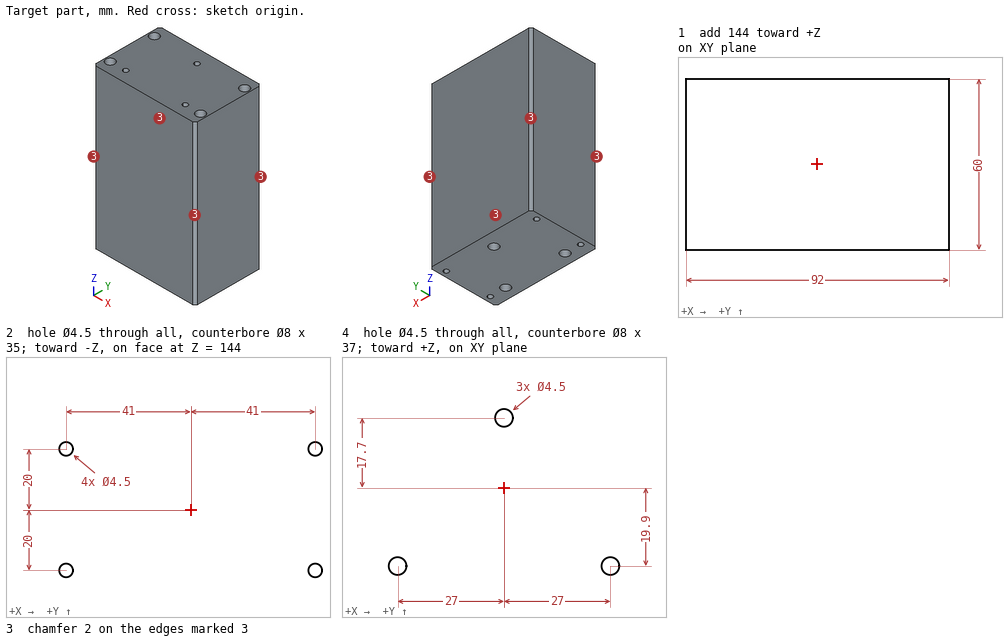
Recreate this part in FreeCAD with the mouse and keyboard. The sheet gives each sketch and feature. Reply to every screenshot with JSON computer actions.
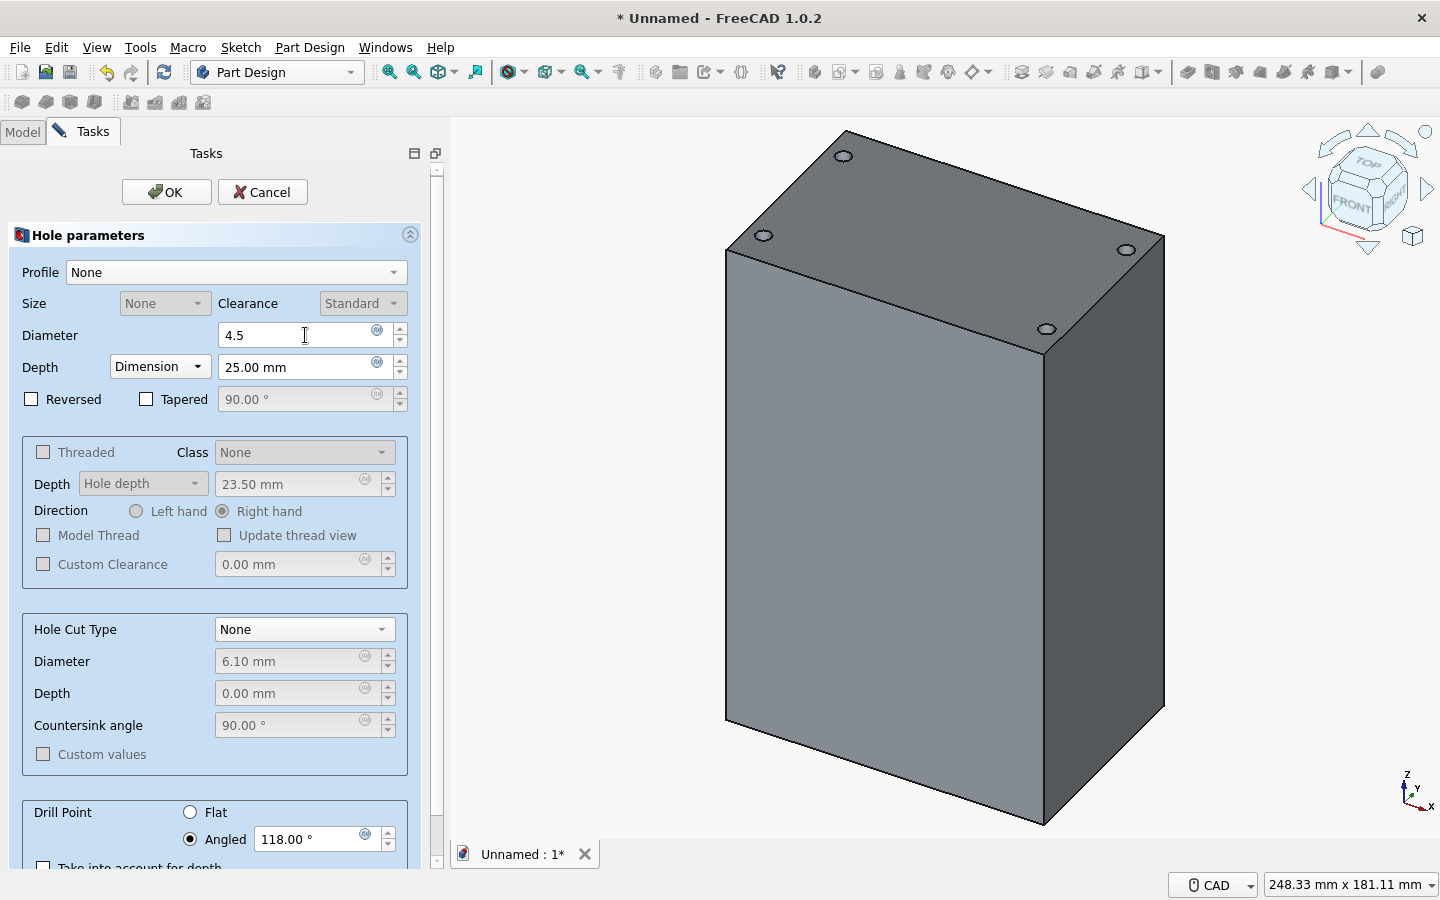
{"action": "left_click", "coordinate": [161, 366]}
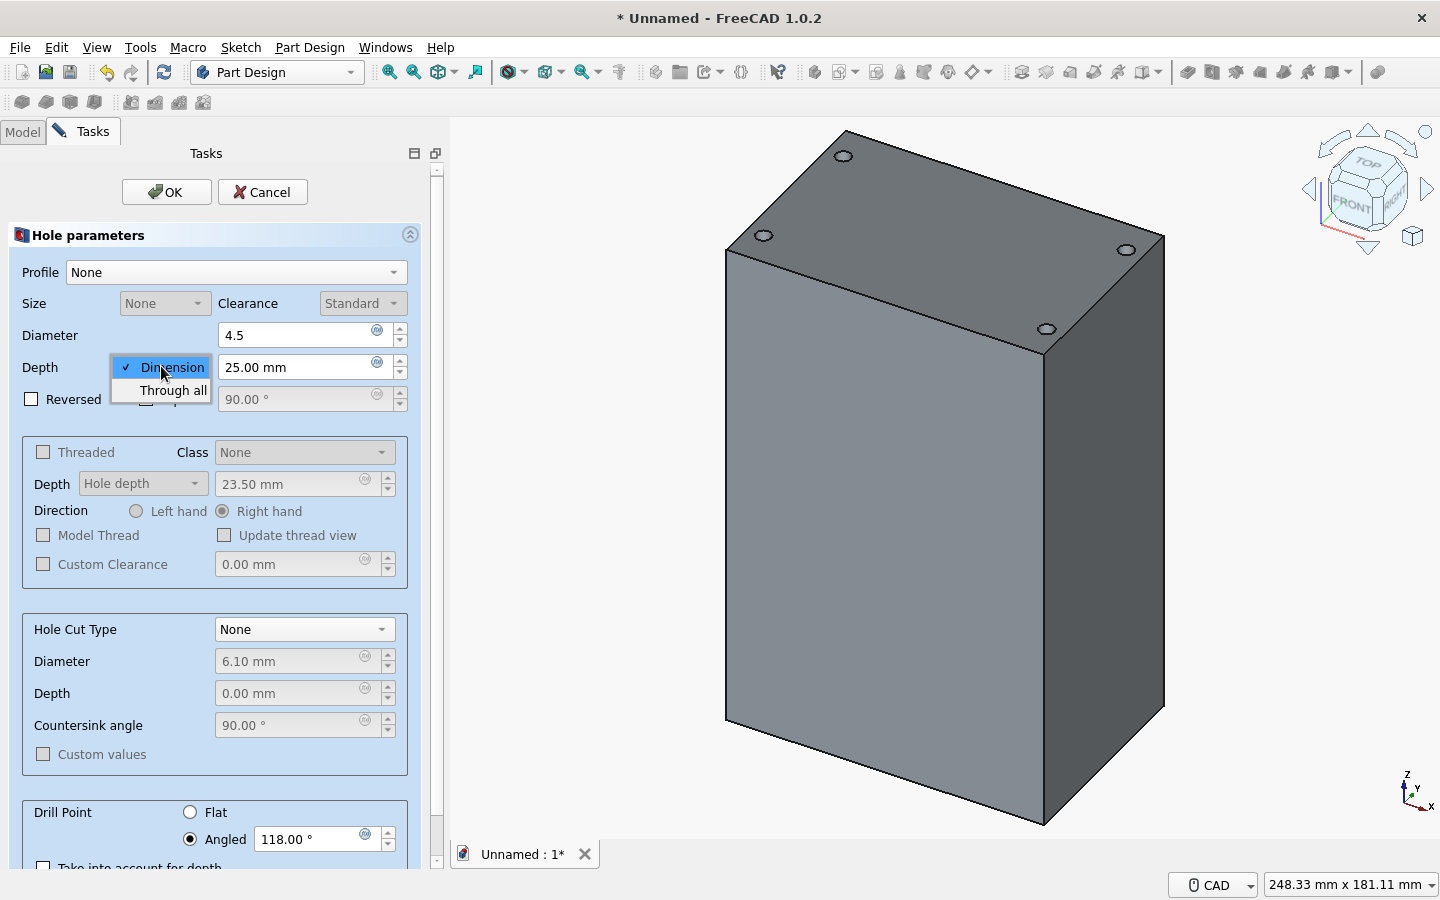
{"action": "left_click", "coordinate": [160, 390]}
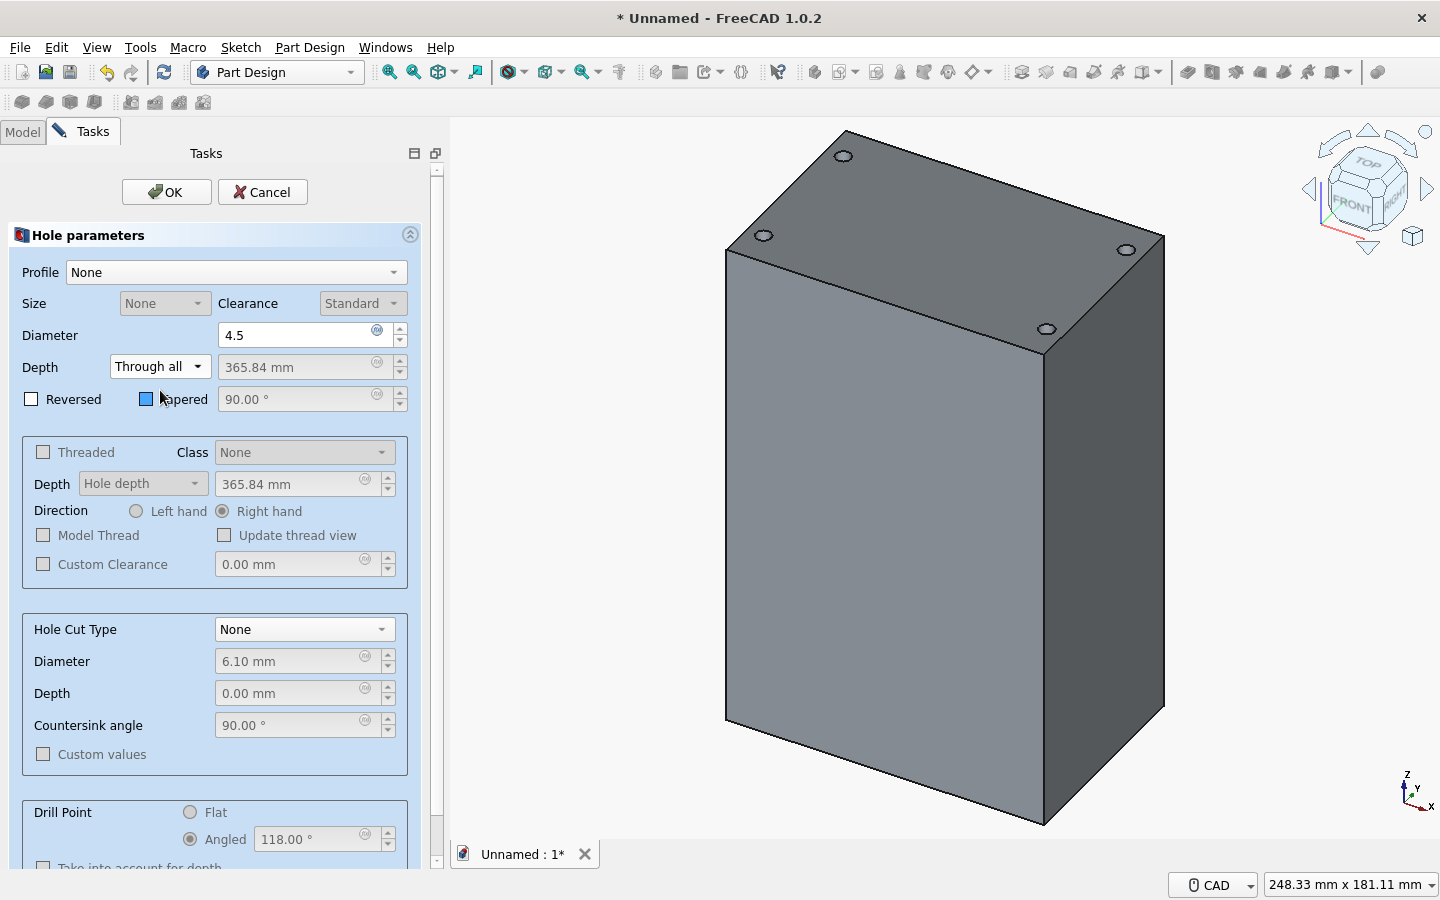
{"action": "left_click", "coordinate": [306, 630]}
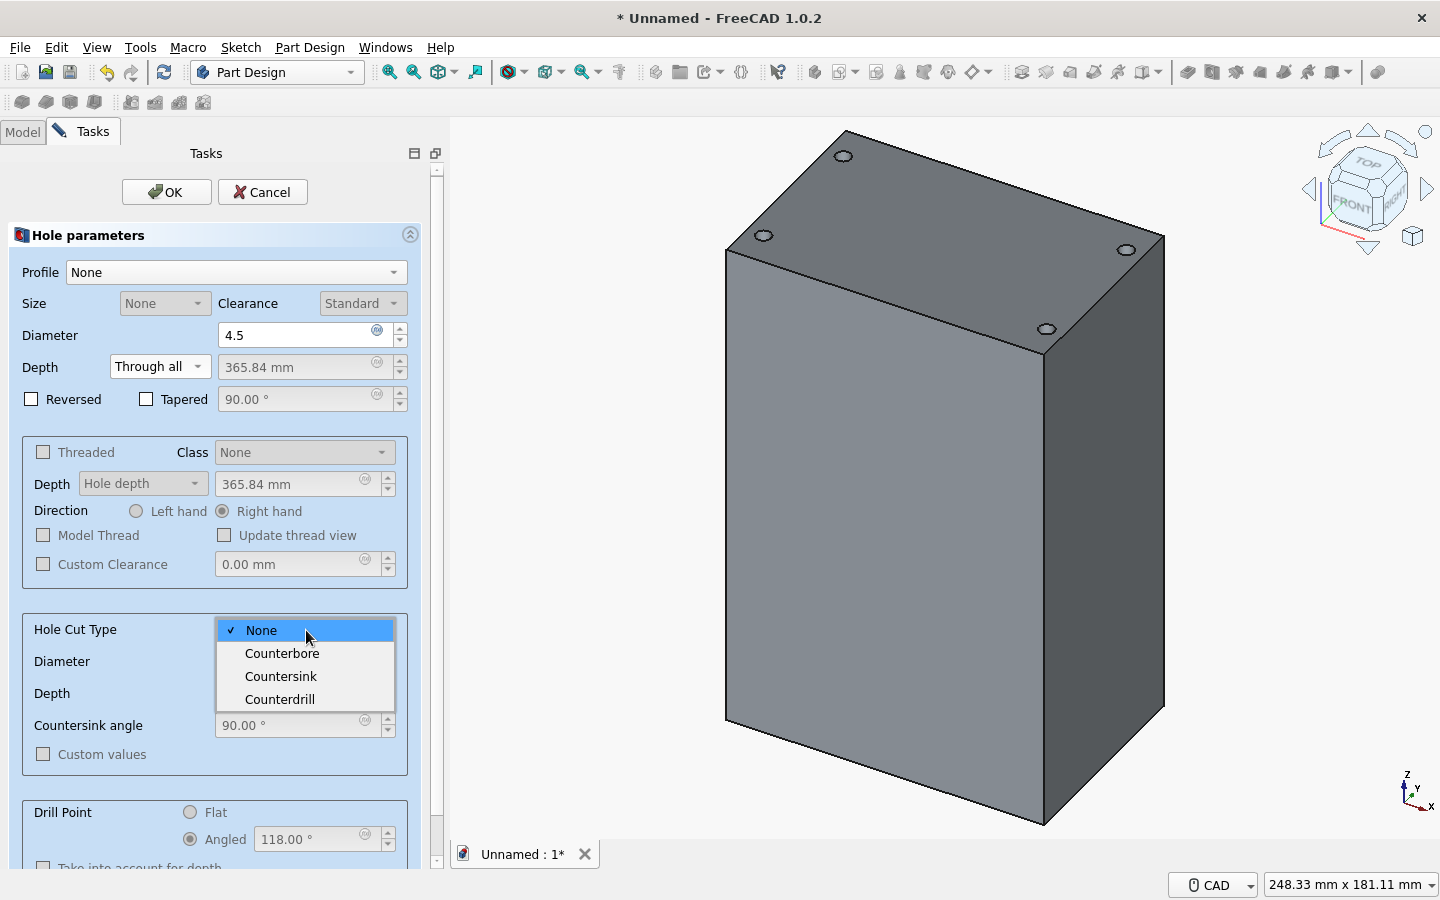
{"action": "left_click", "coordinate": [304, 654]}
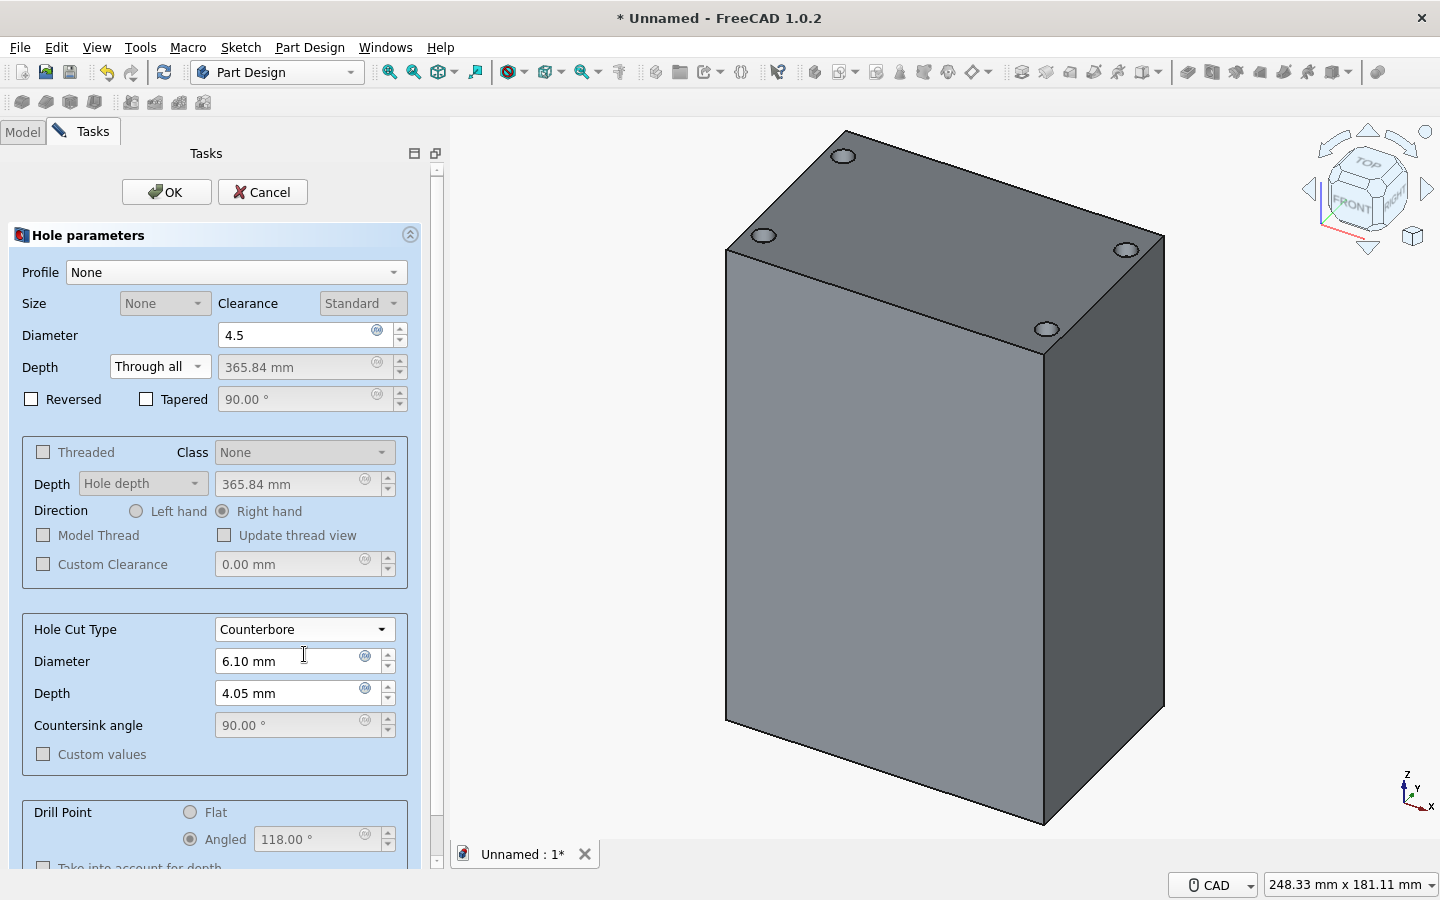
{"action": "triple_click", "coordinate": [298, 661]}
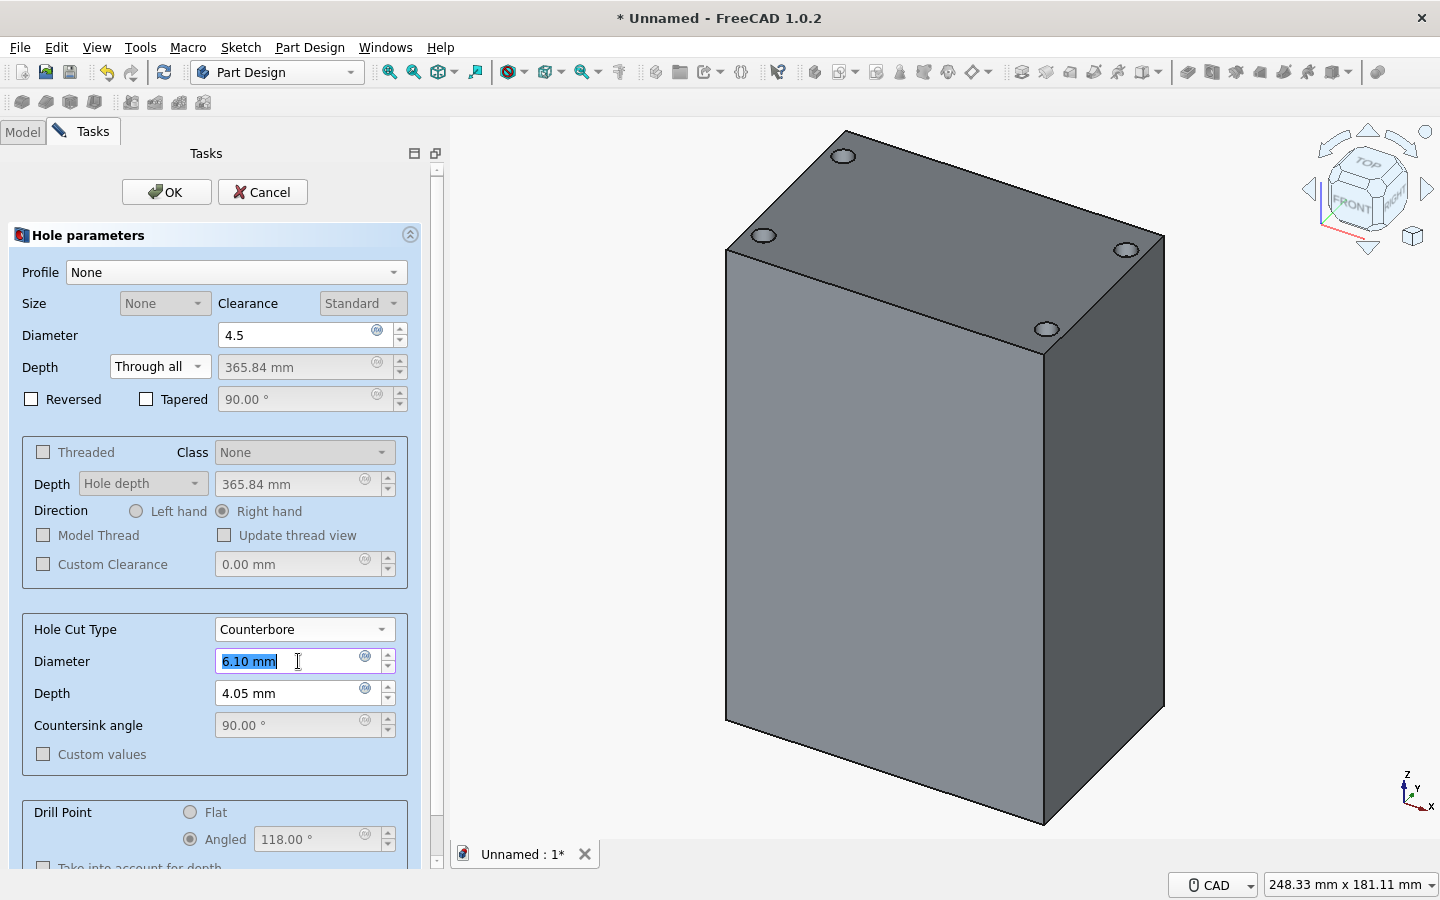
{"action": "type", "text": "8"}
{"action": "key", "text": "Tab"}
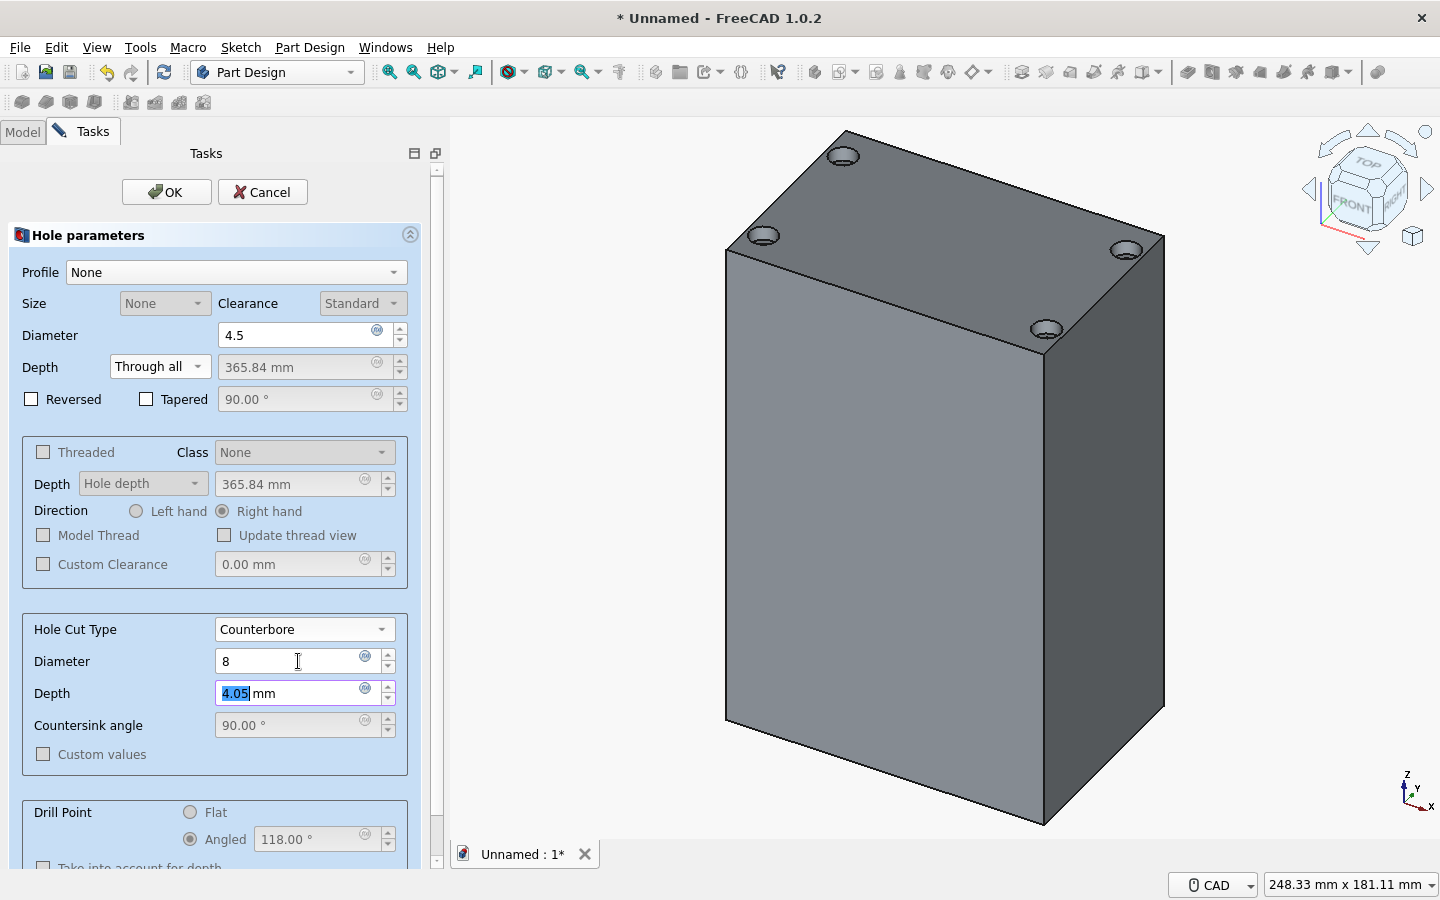
{"action": "type", "text": "35"}
{"action": "key", "text": "Tab"}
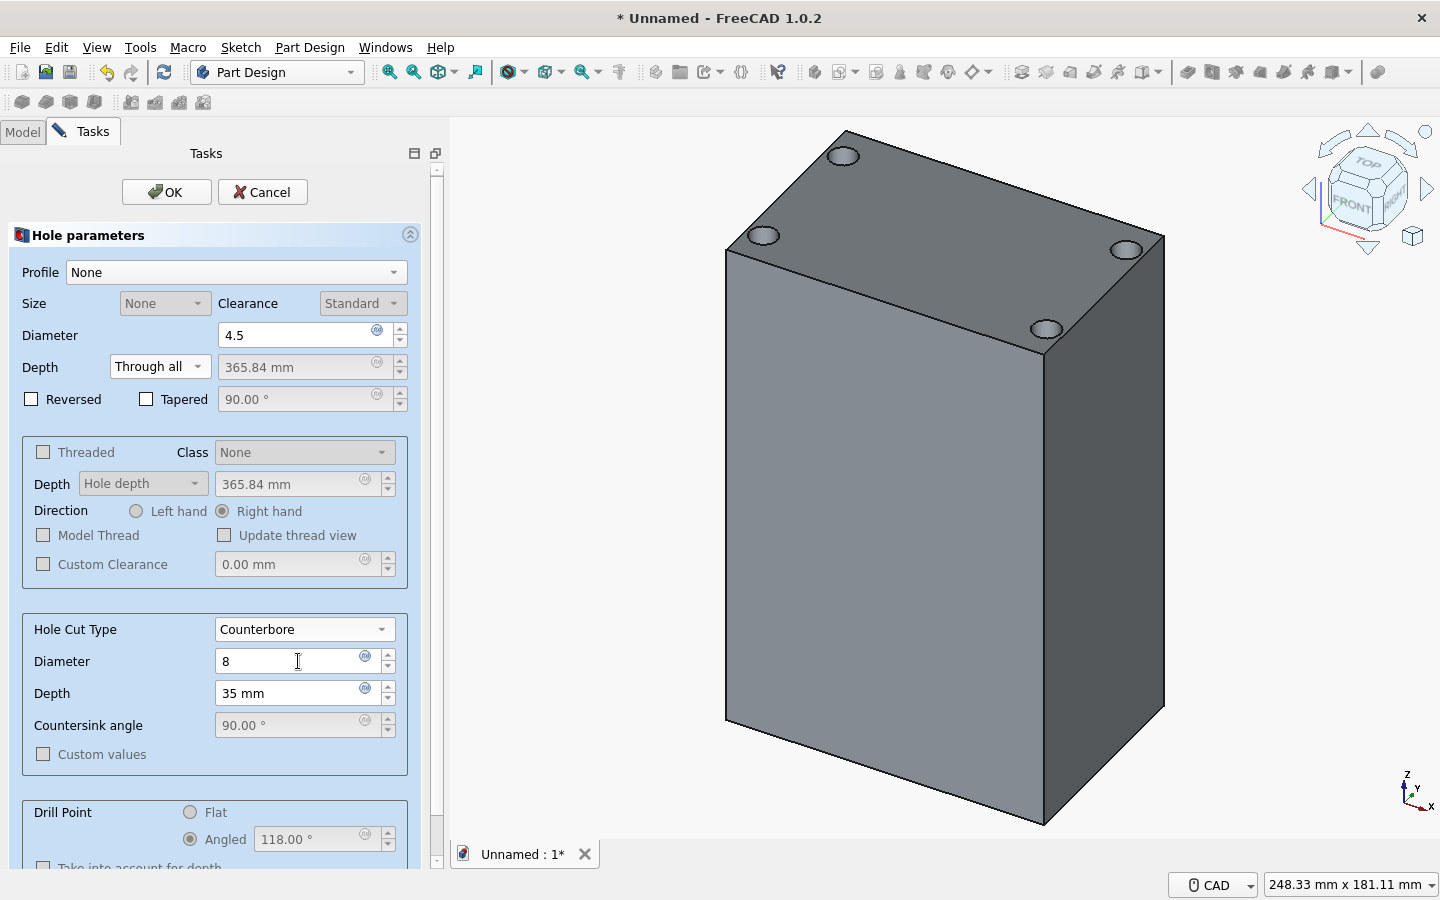
{"action": "left_click", "coordinate": [167, 192]}